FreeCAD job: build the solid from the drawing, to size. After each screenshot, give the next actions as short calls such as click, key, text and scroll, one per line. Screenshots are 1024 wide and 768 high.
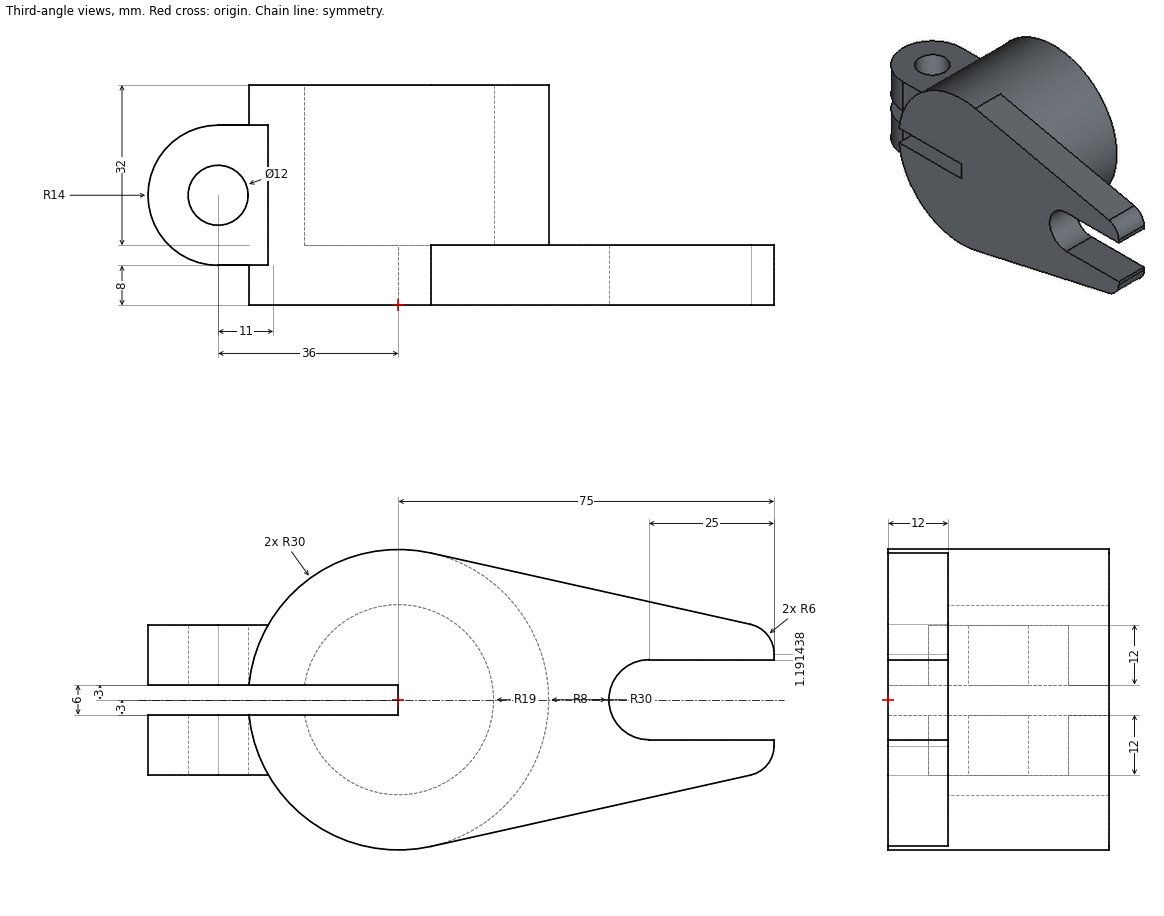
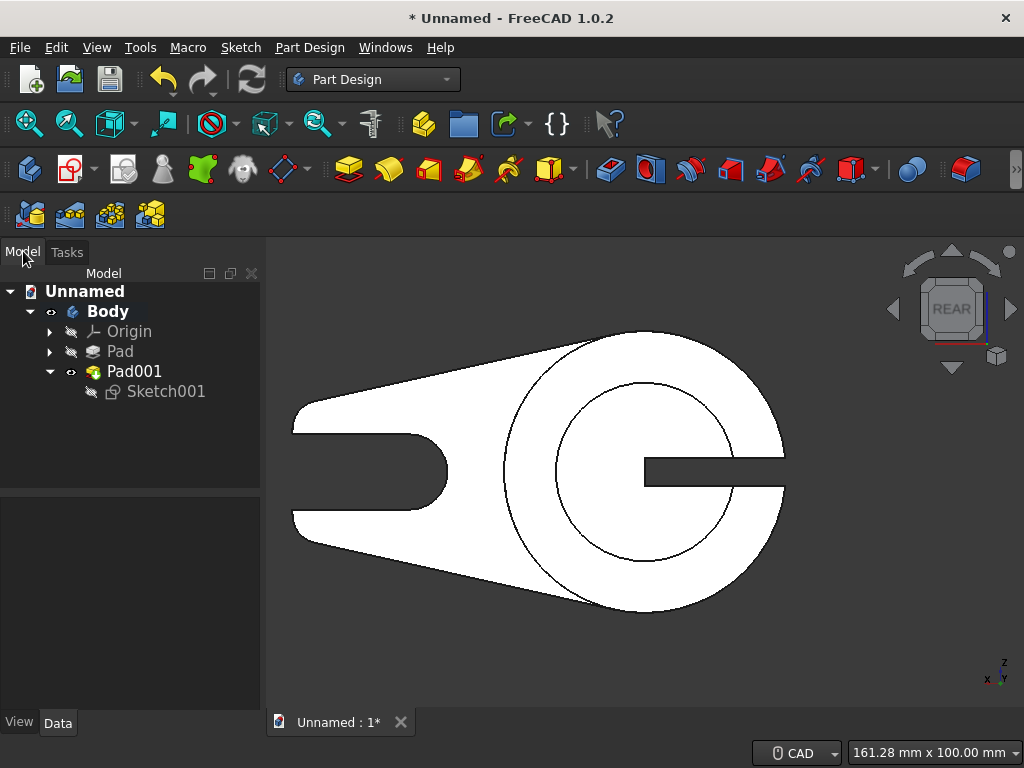
click(50, 332)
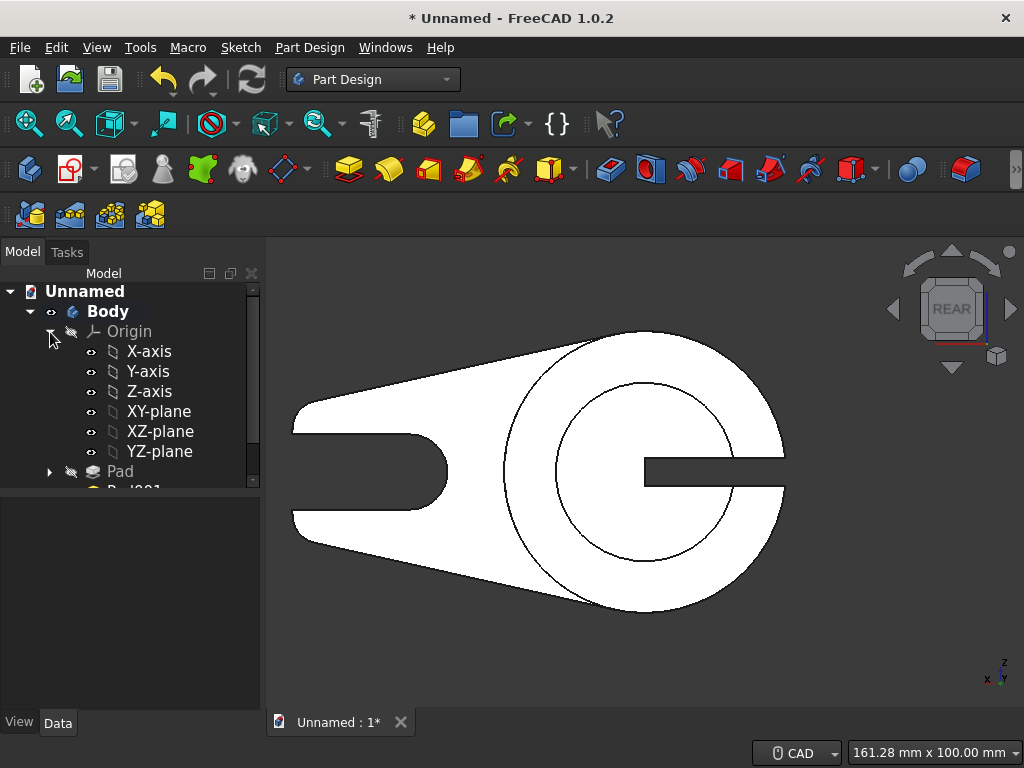
click(136, 412)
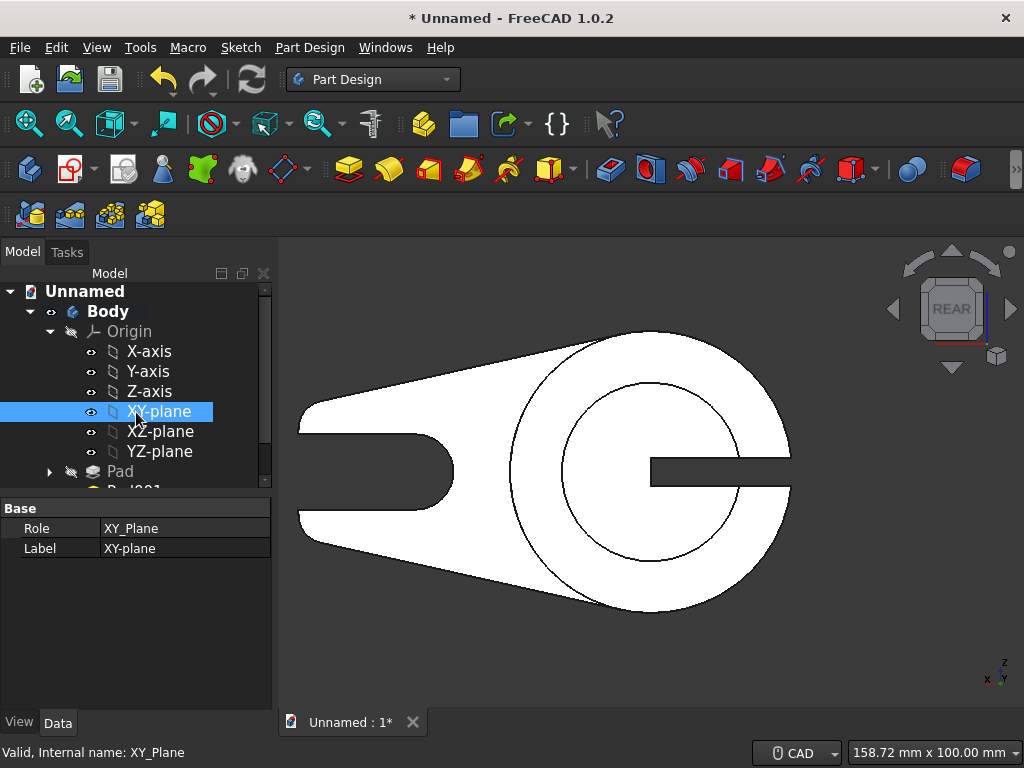
click(284, 170)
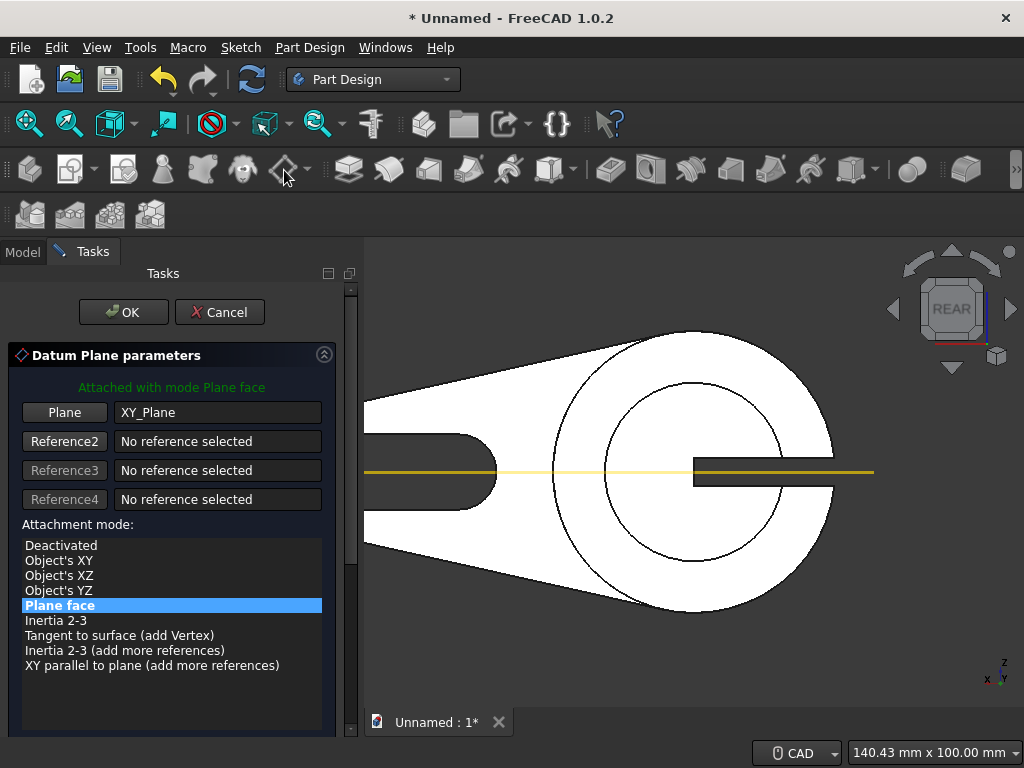
scroll(351, 510, down, 3)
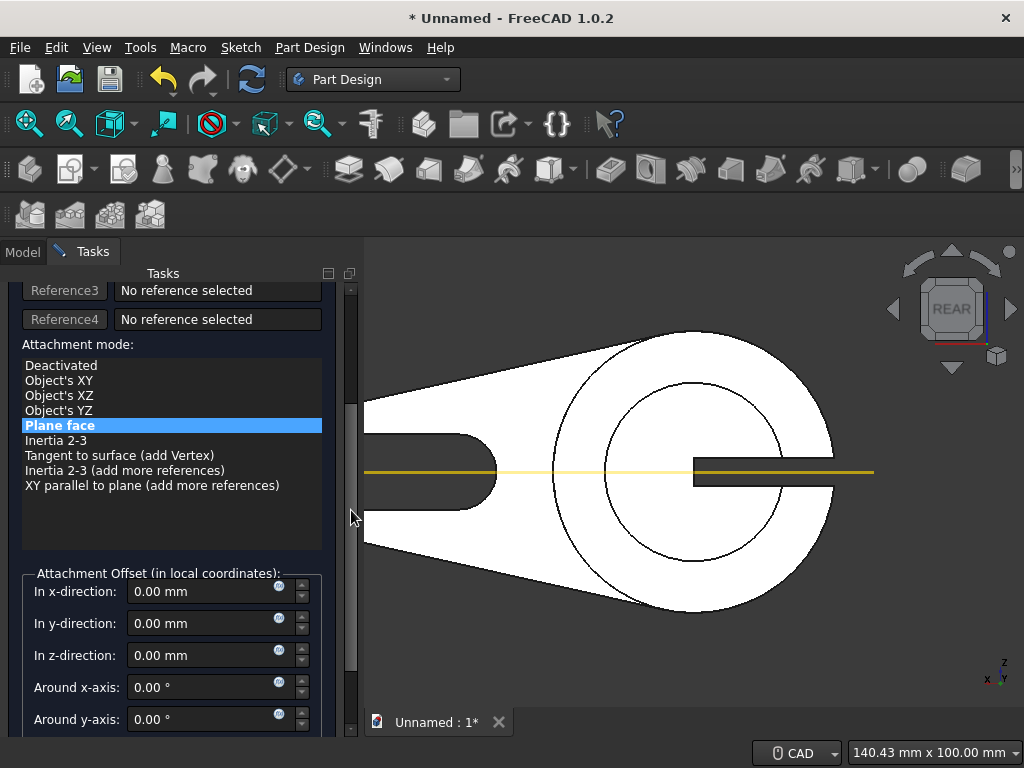
triple_click(210, 655)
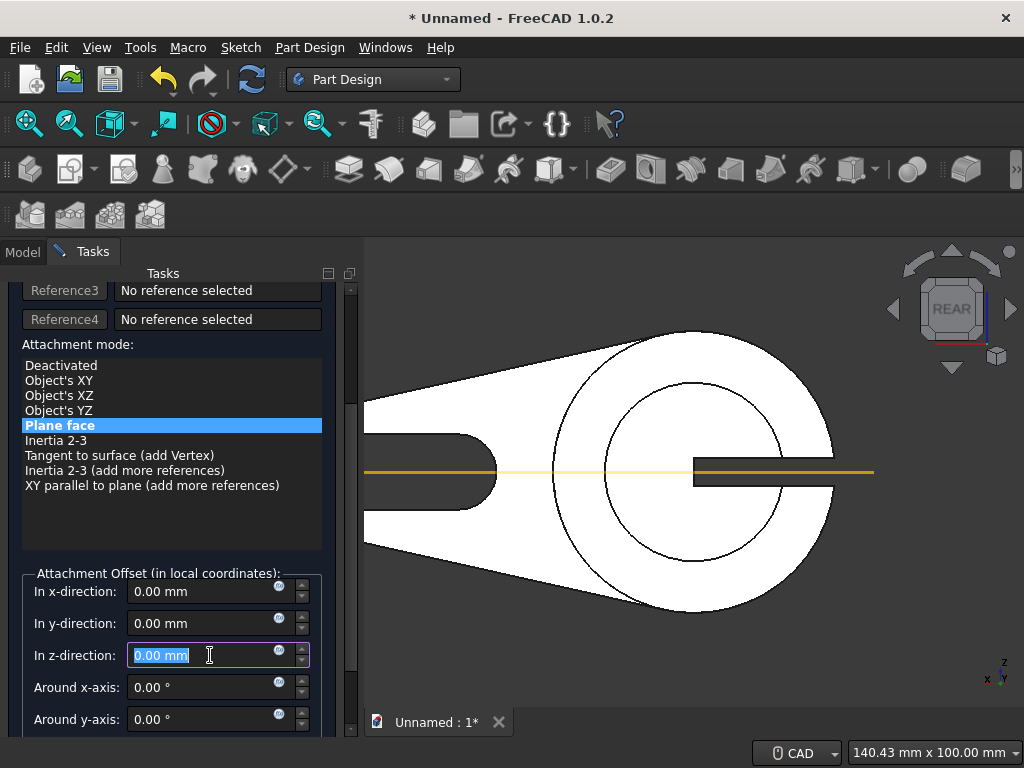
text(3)
key(Tab)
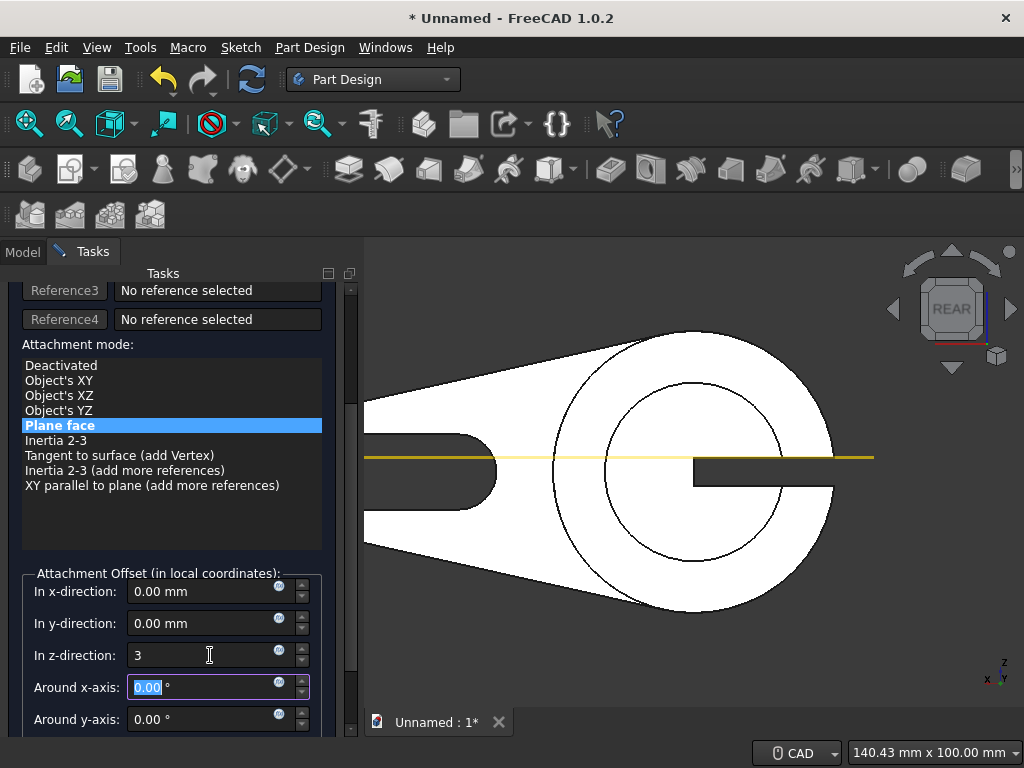
scroll(351, 510, up, 4)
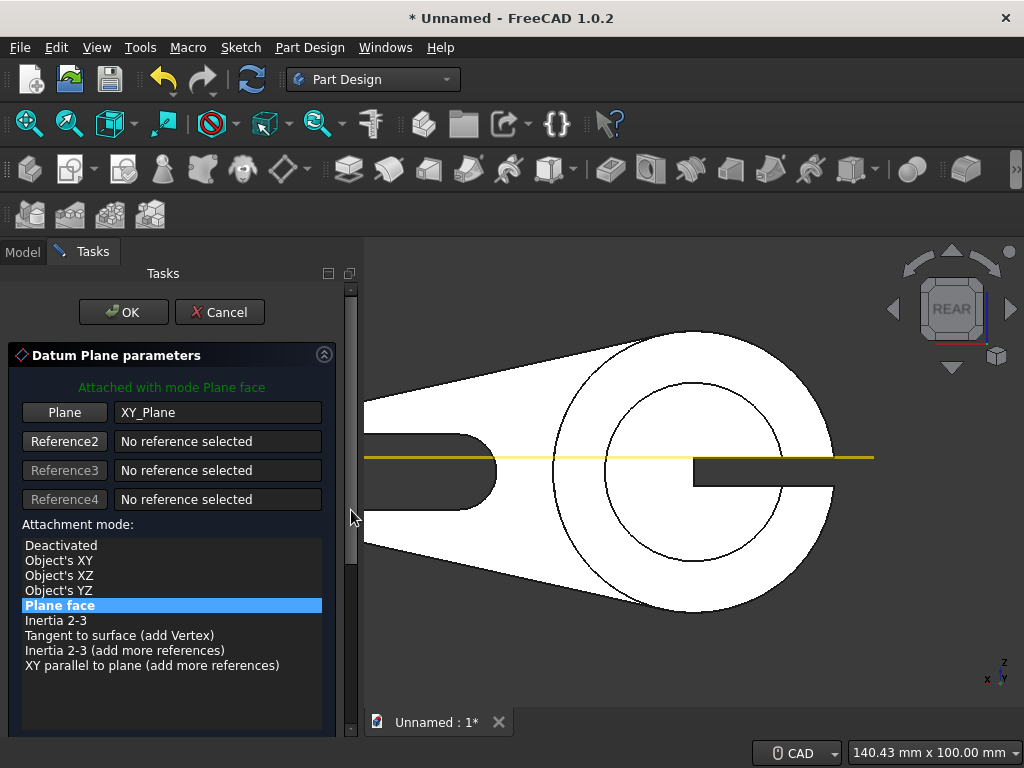
click(124, 312)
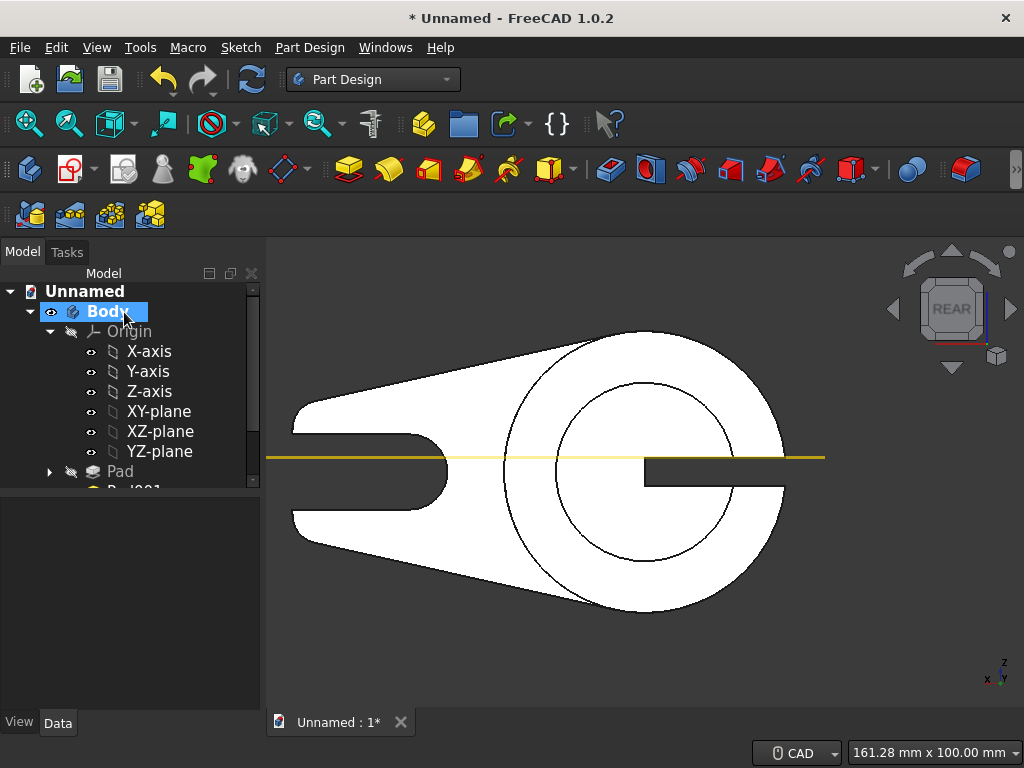
scroll(100, 387, down, 3)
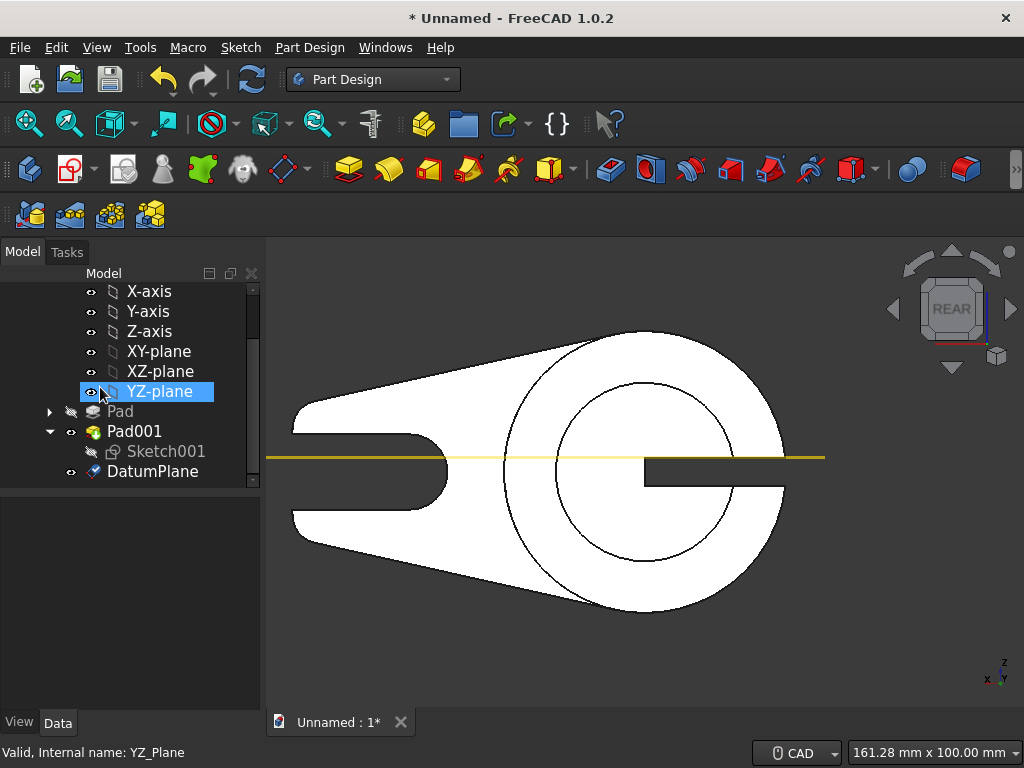
click(116, 472)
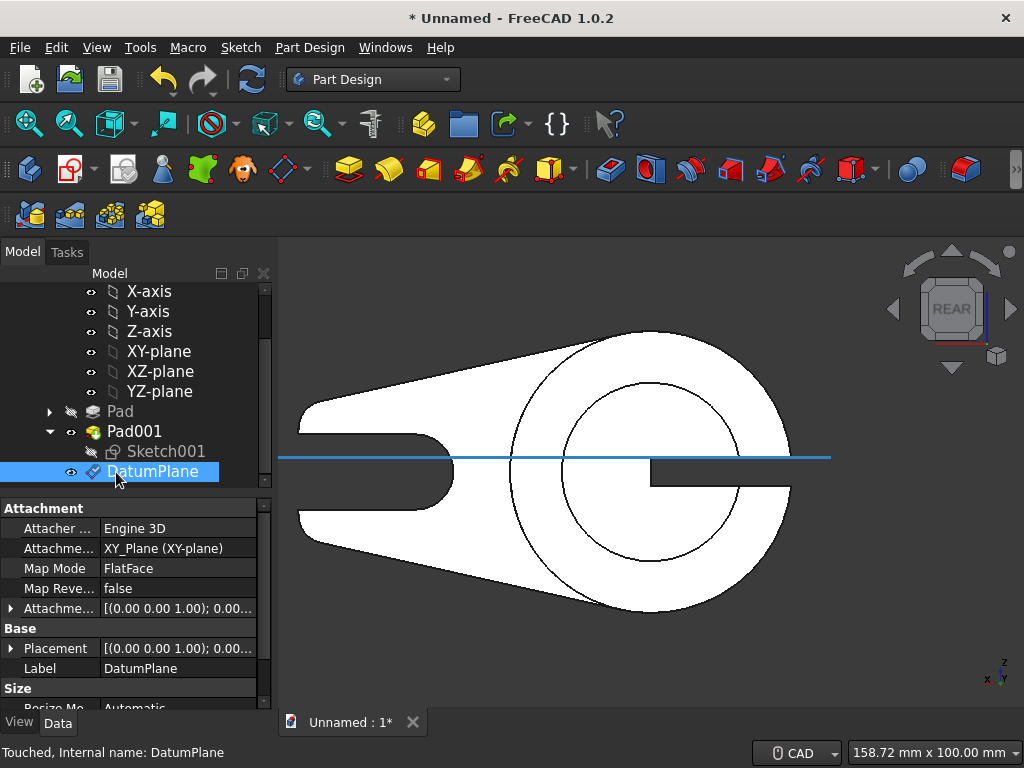
click(70, 170)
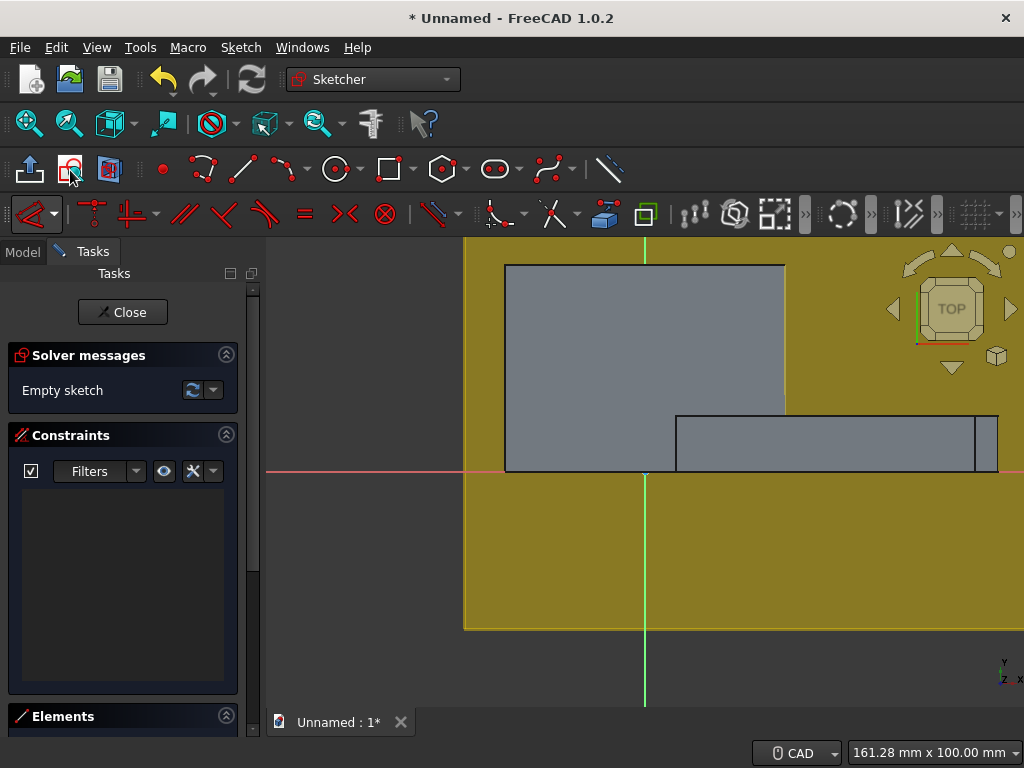
key(q)
key(s)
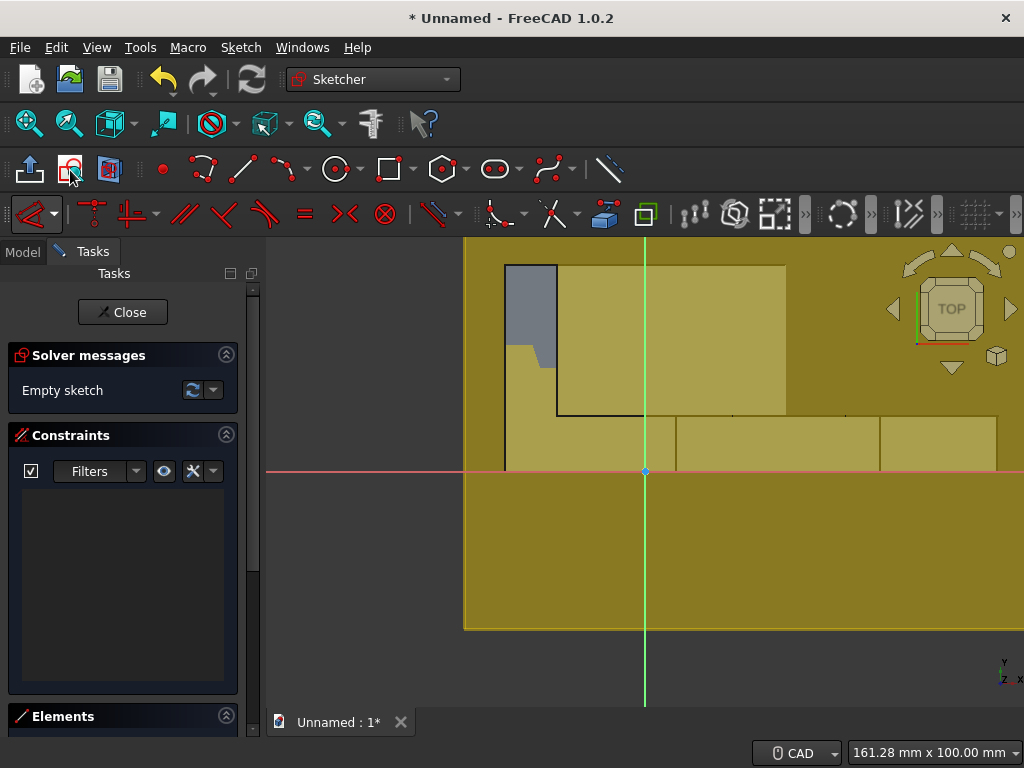
scroll(468, 284, up, 3)